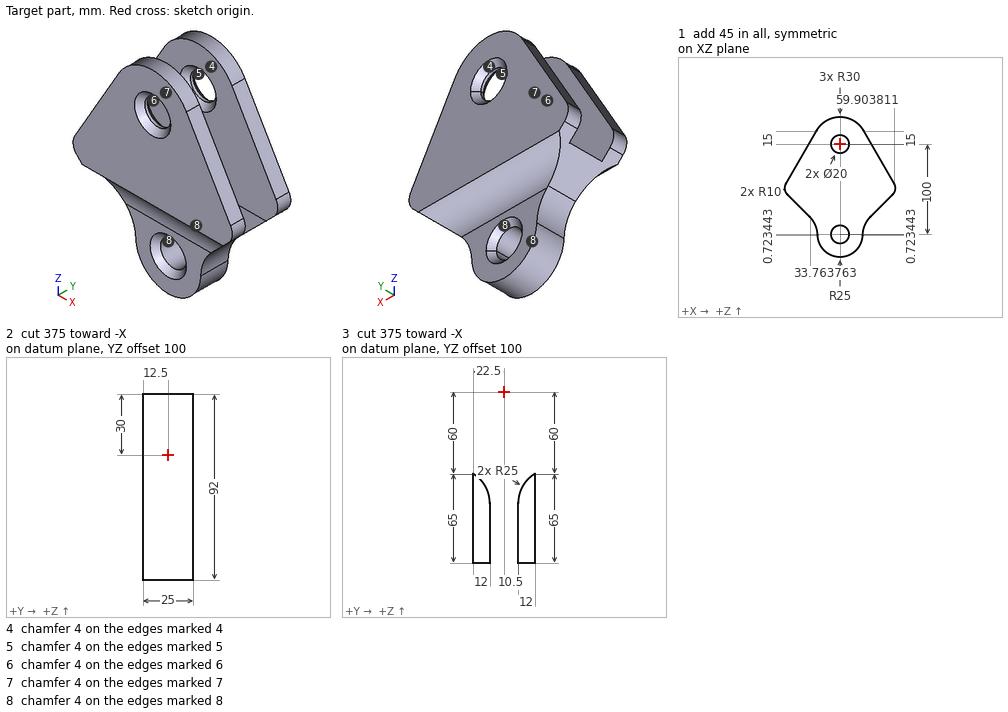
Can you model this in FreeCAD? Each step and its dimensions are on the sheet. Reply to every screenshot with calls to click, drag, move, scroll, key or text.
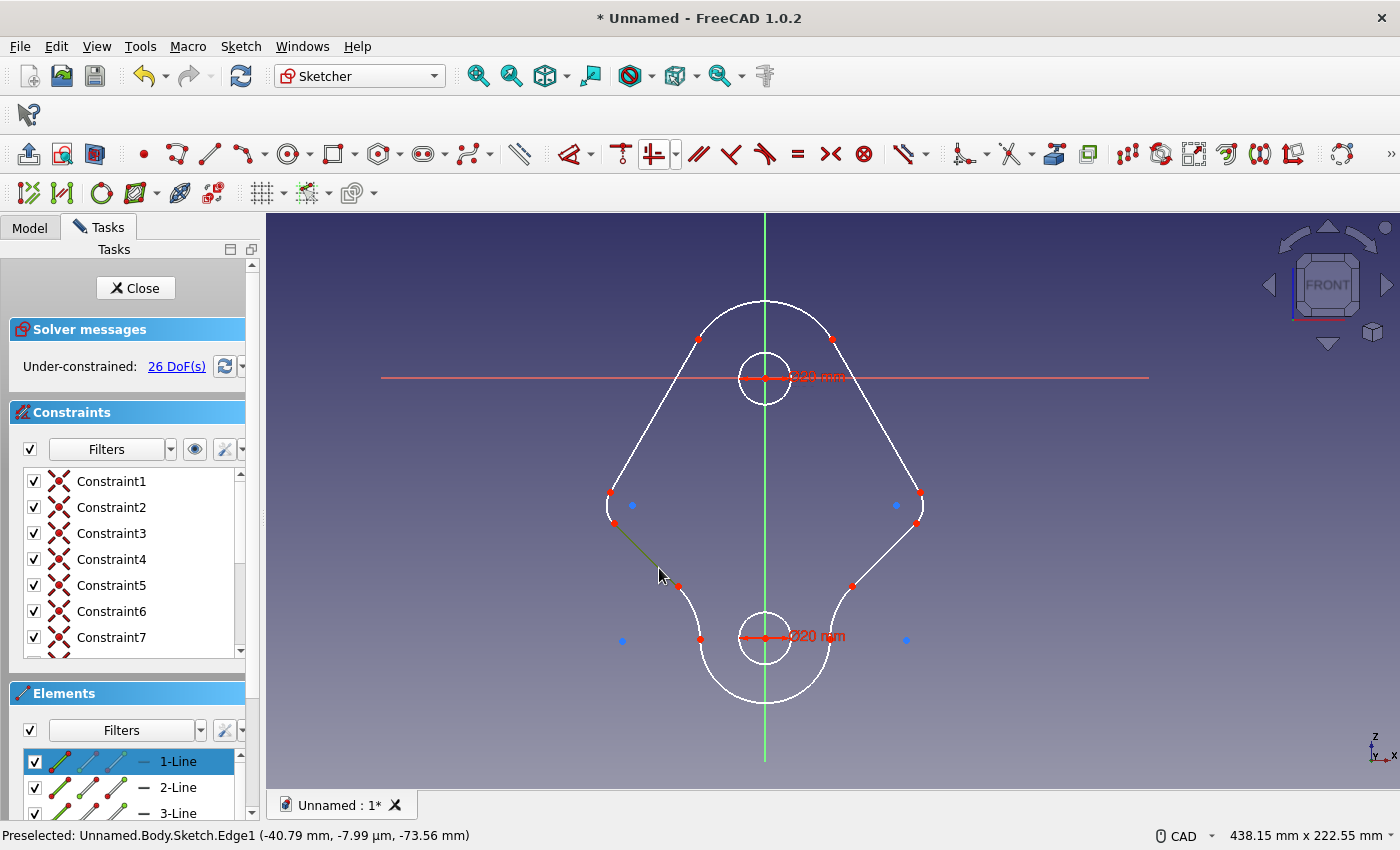
scroll(607, 502, up, 2)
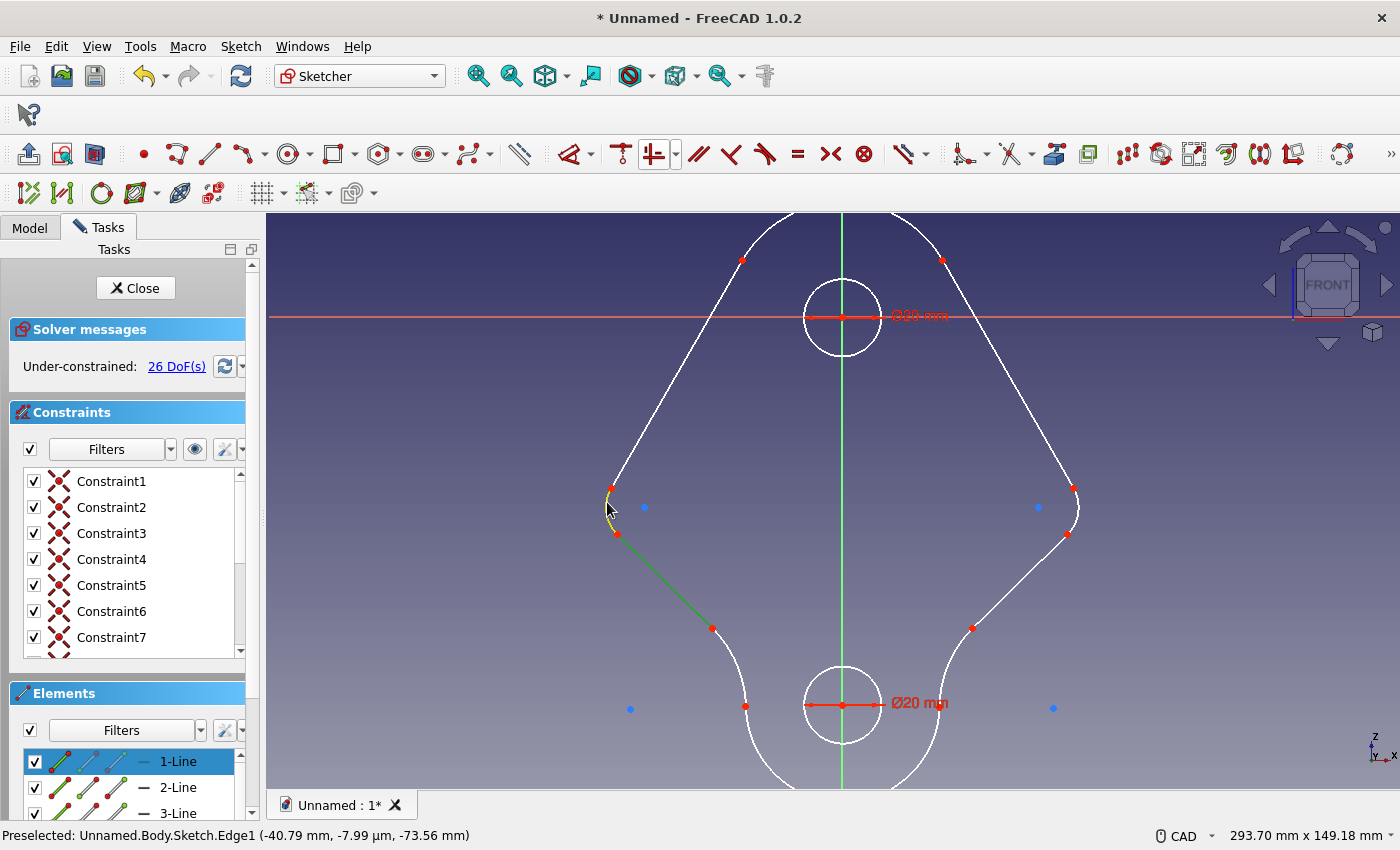
click(606, 502)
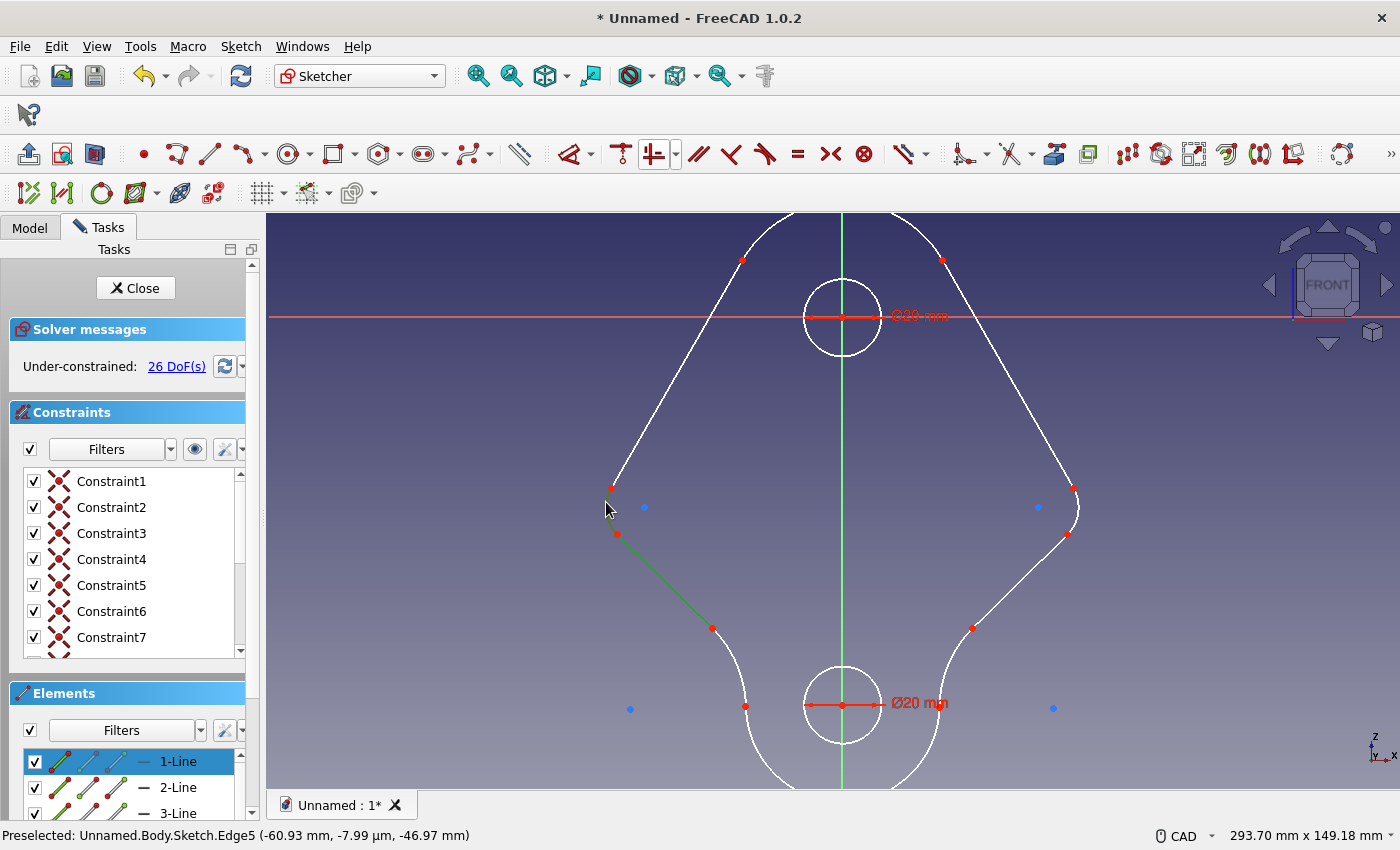
click(765, 154)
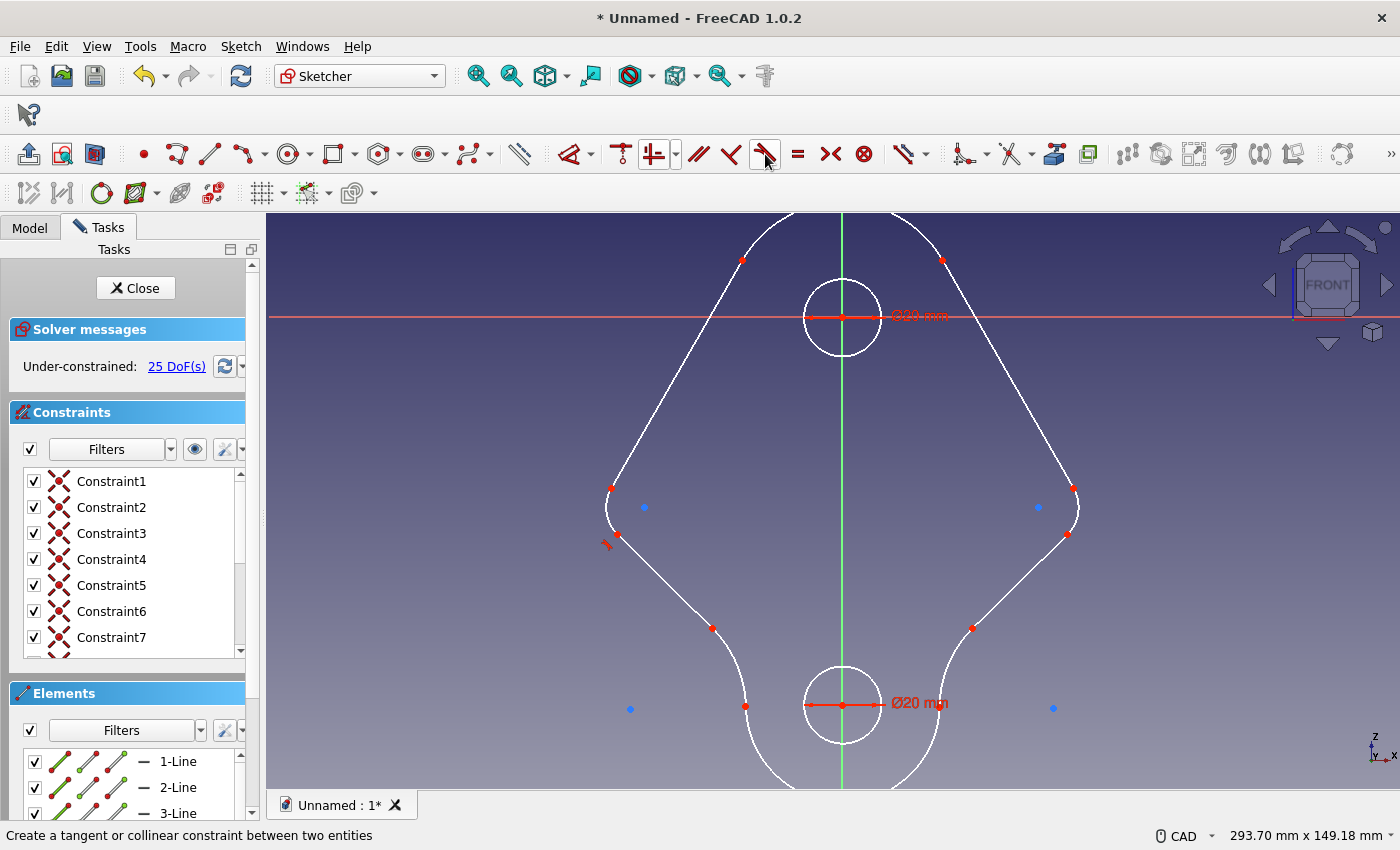
click(684, 600)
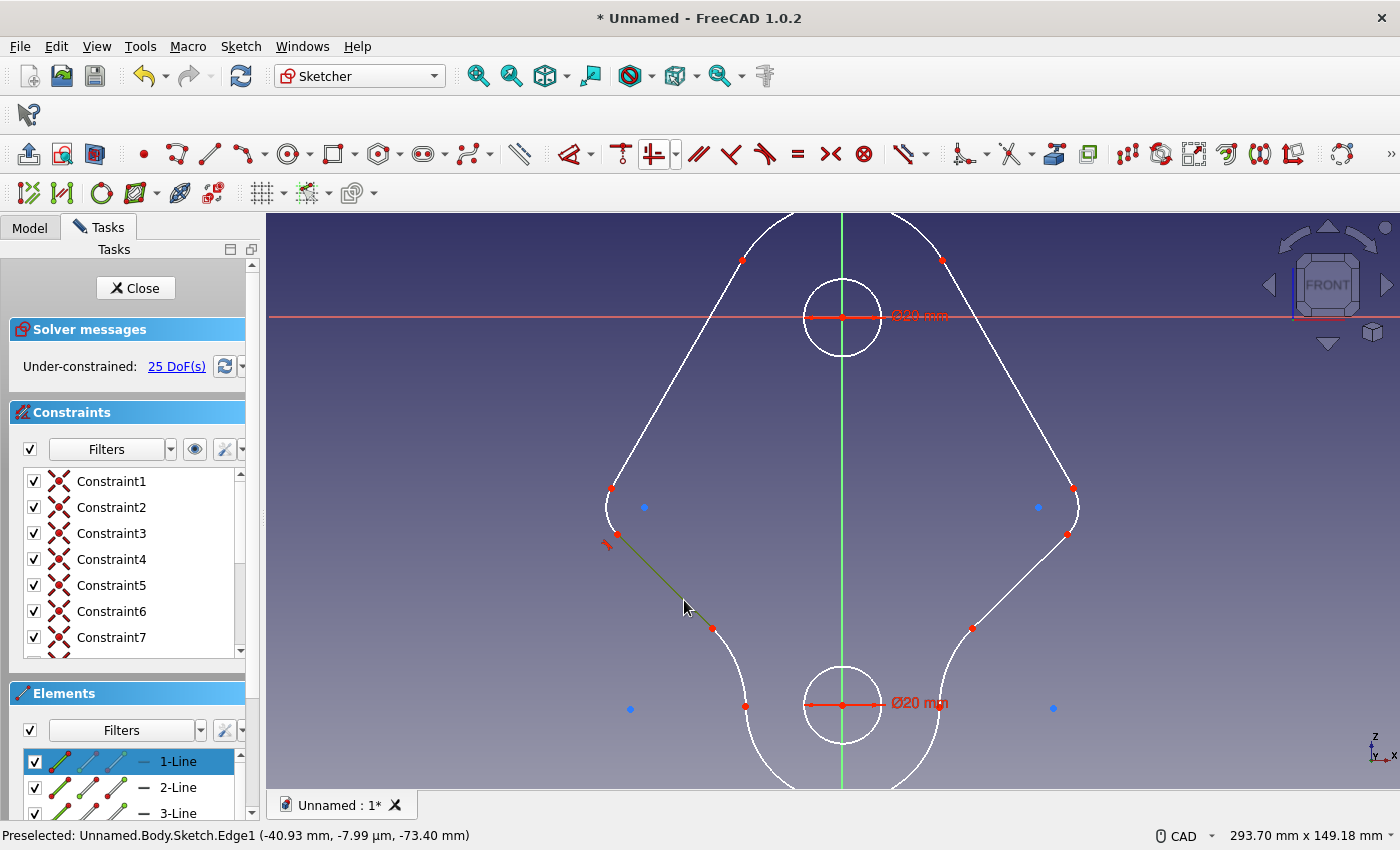
click(742, 681)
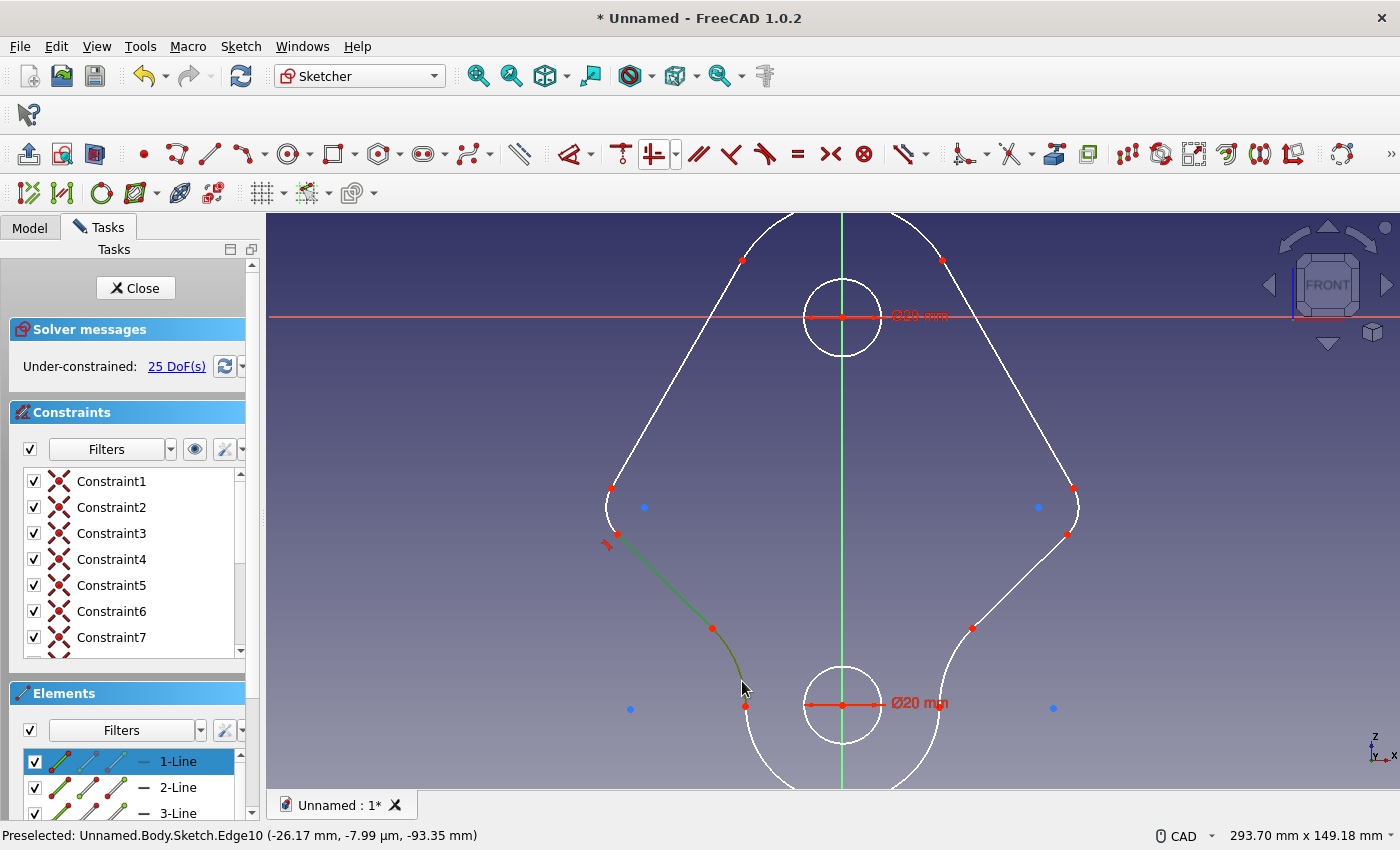
click(765, 154)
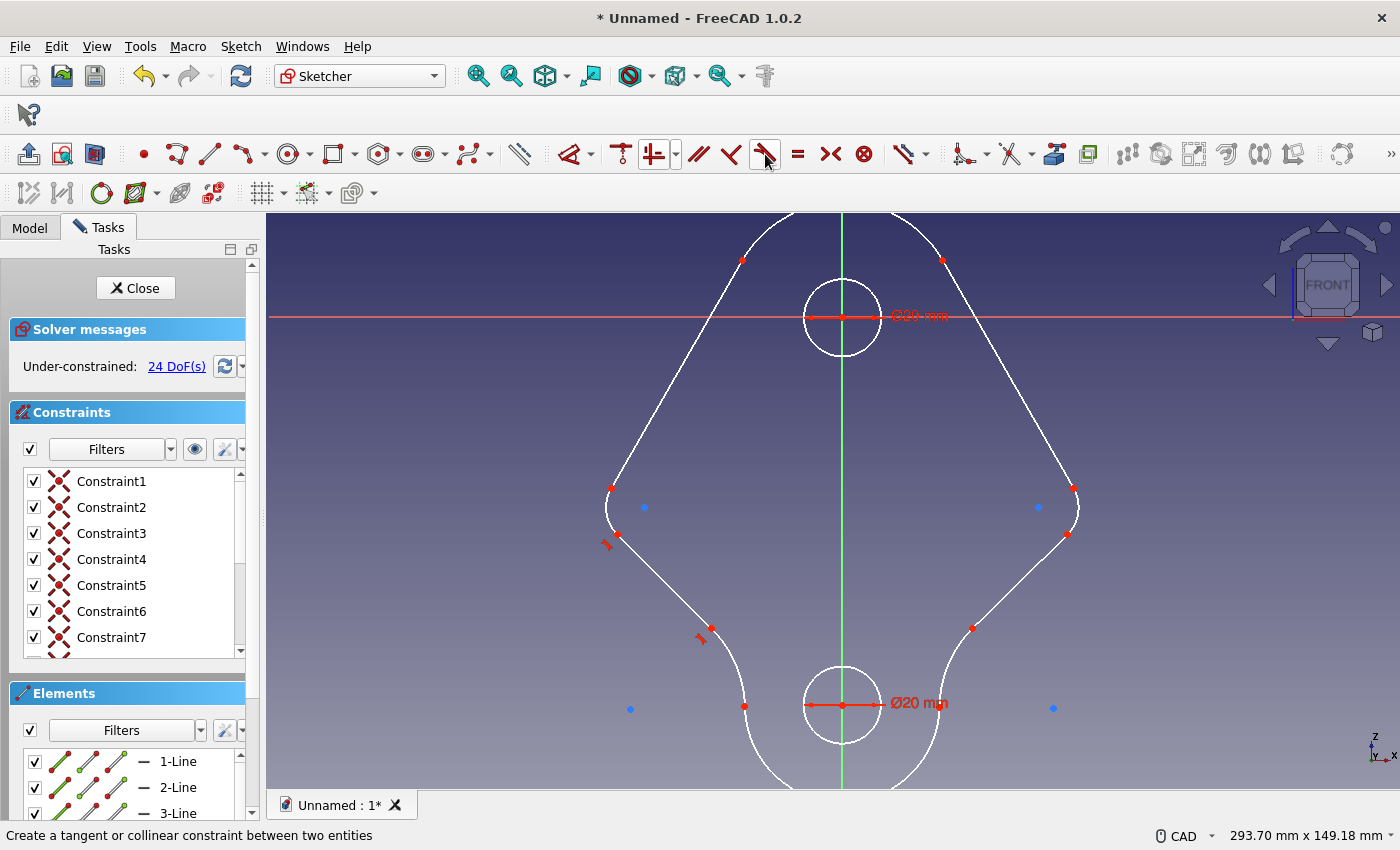
click(651, 420)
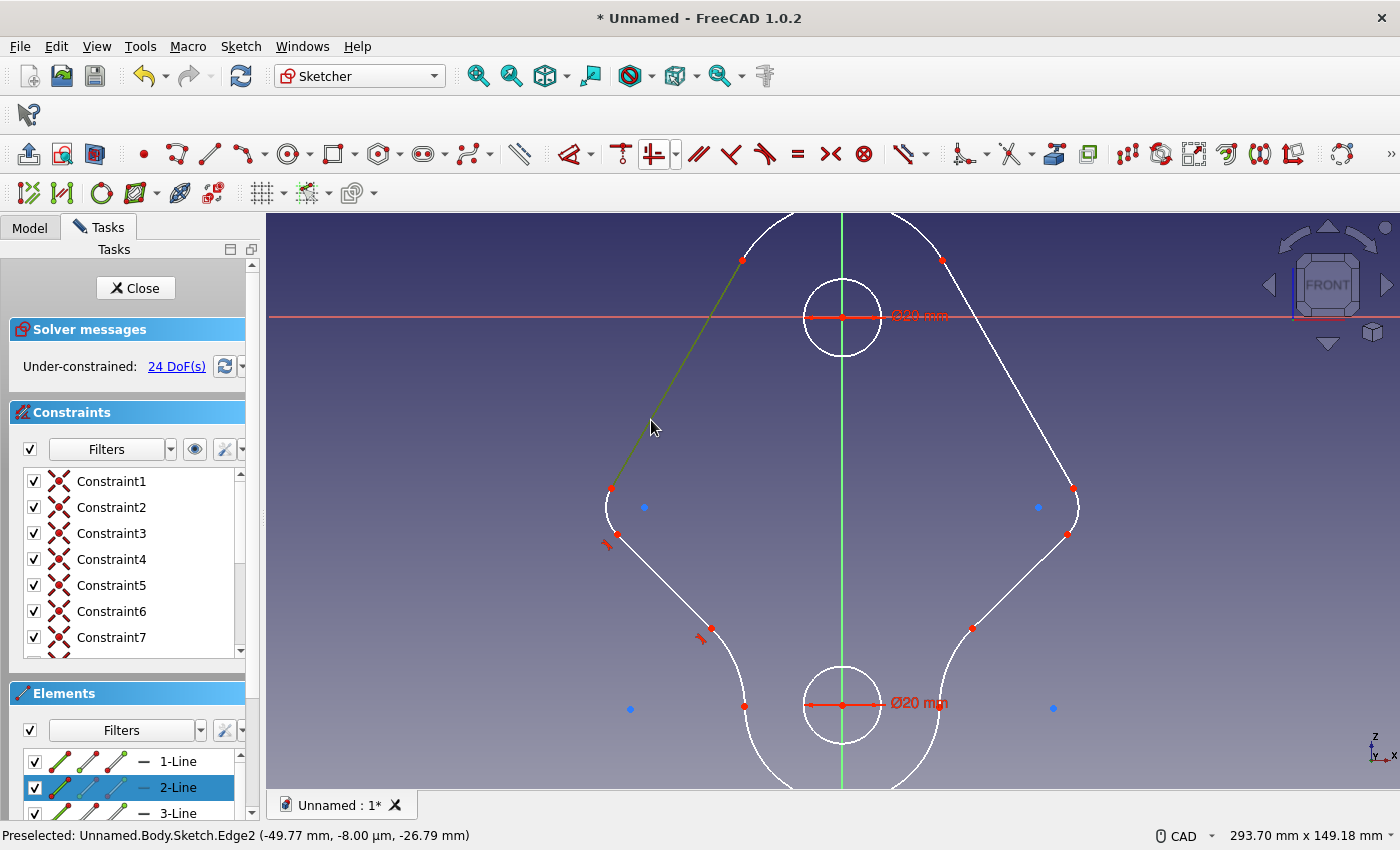
click(606, 502)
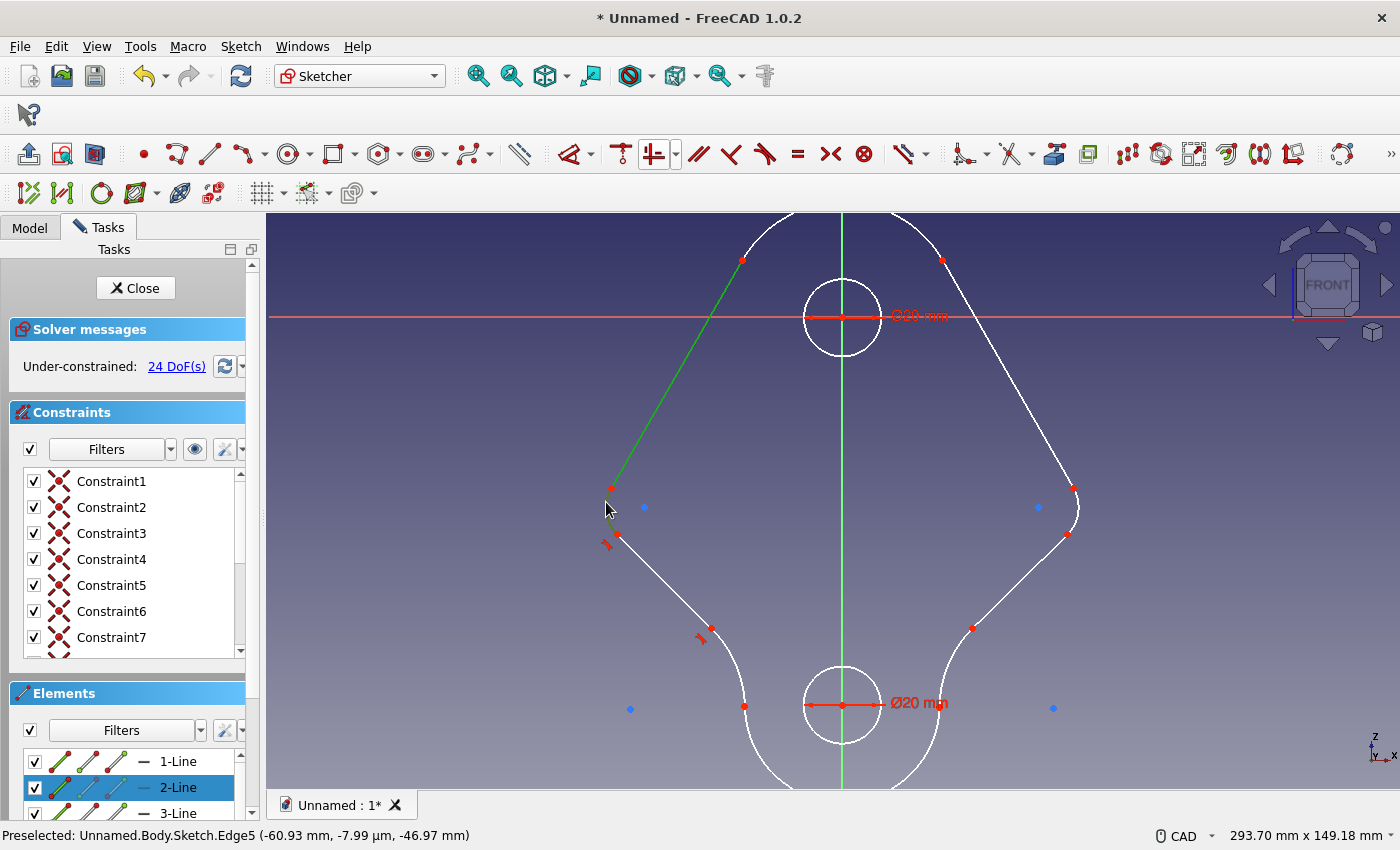
click(765, 154)